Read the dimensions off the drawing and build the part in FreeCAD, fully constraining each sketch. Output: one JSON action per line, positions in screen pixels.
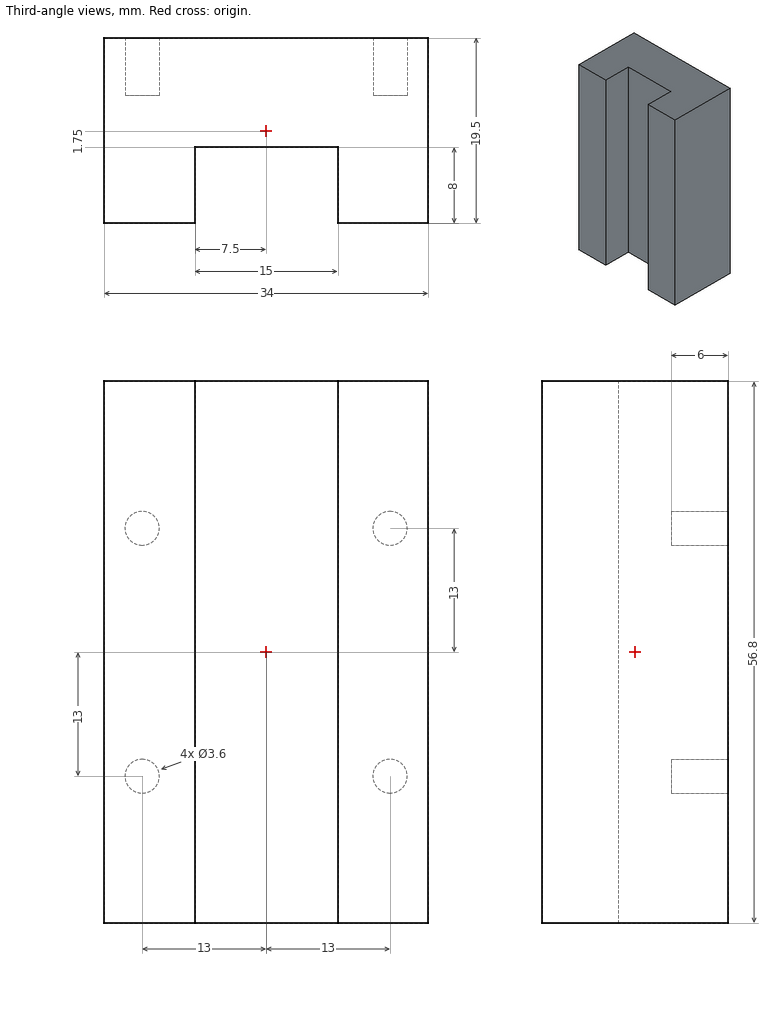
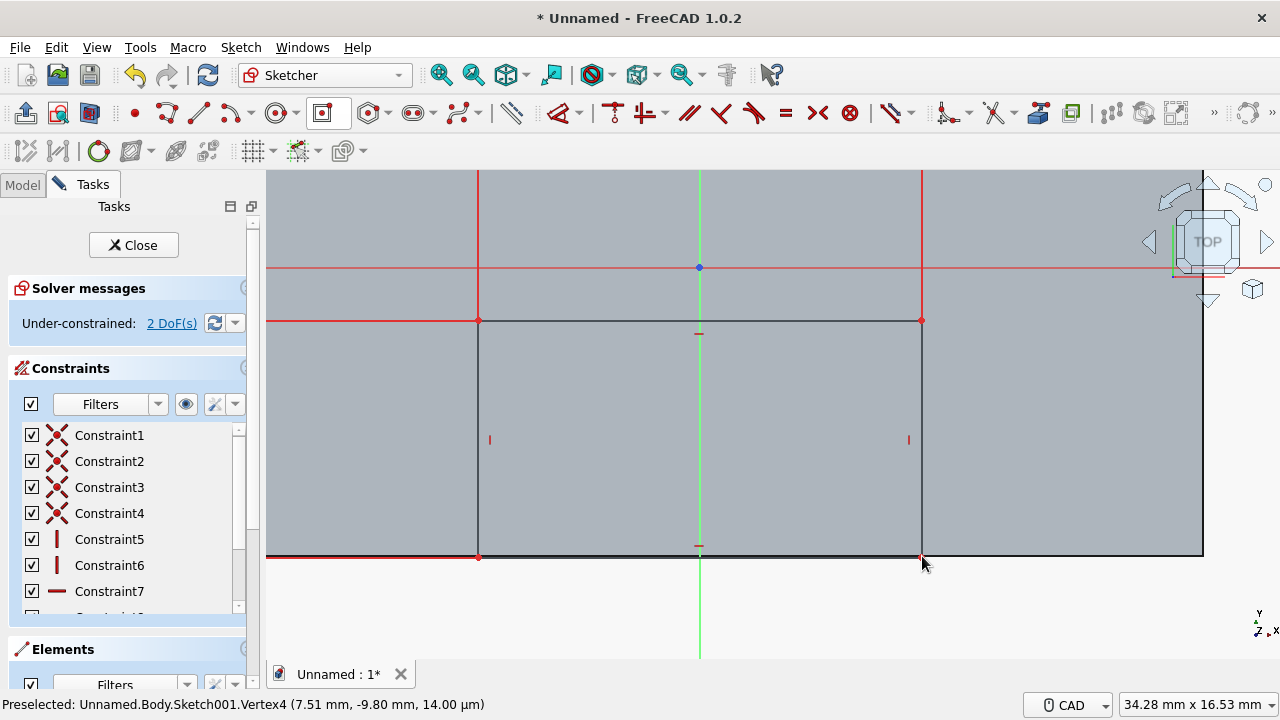
{"action": "left_click", "coordinate": [478, 321]}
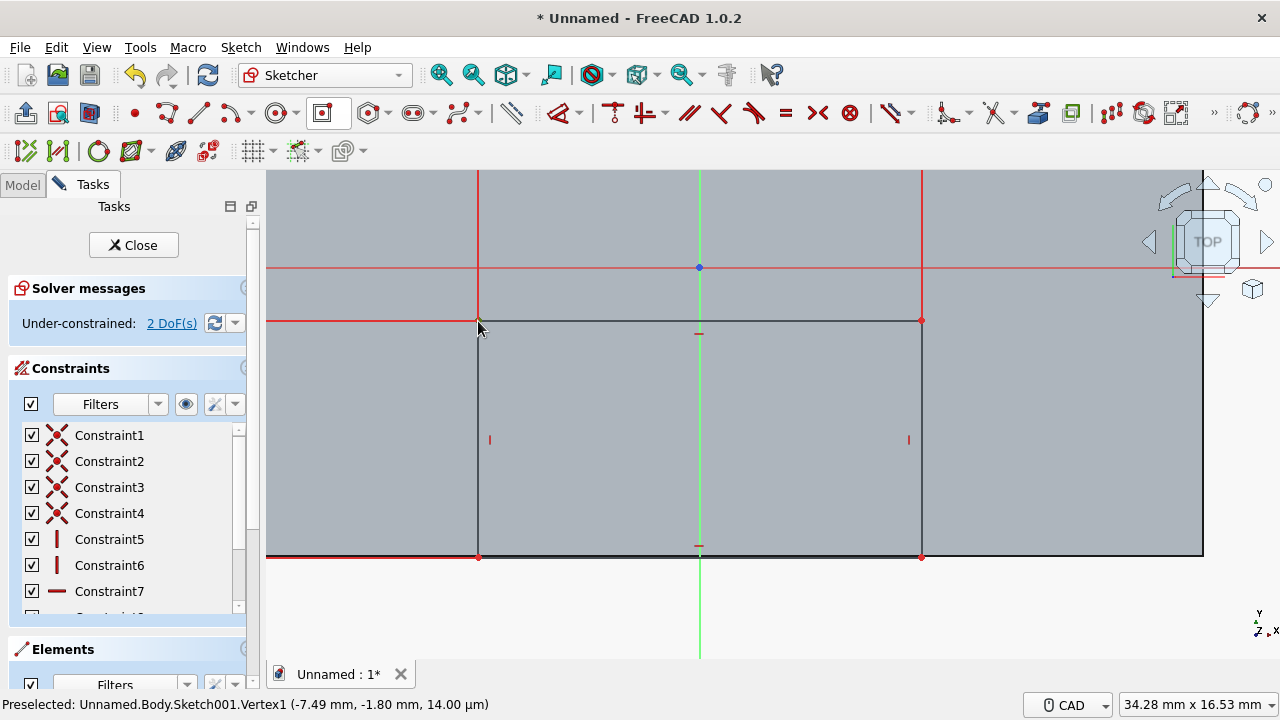
{"action": "key", "text": "l"}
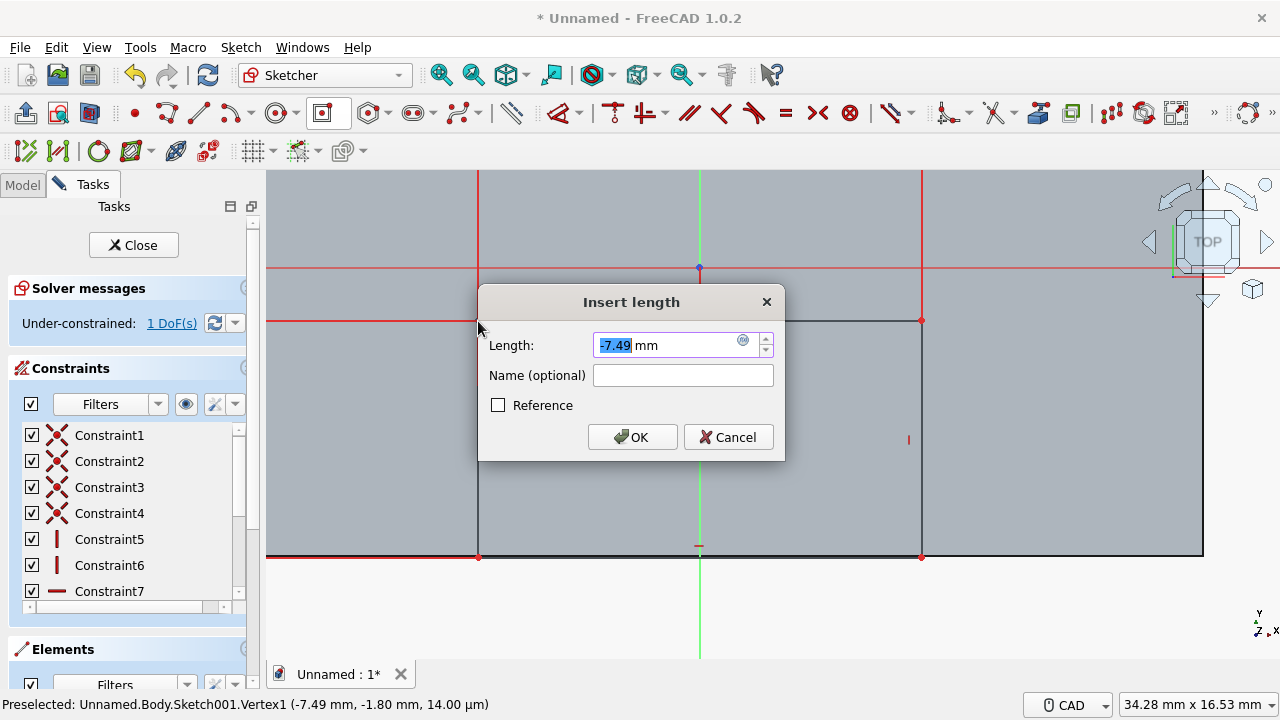
{"action": "type", "text": "-7.5"}
{"action": "key", "text": "Return"}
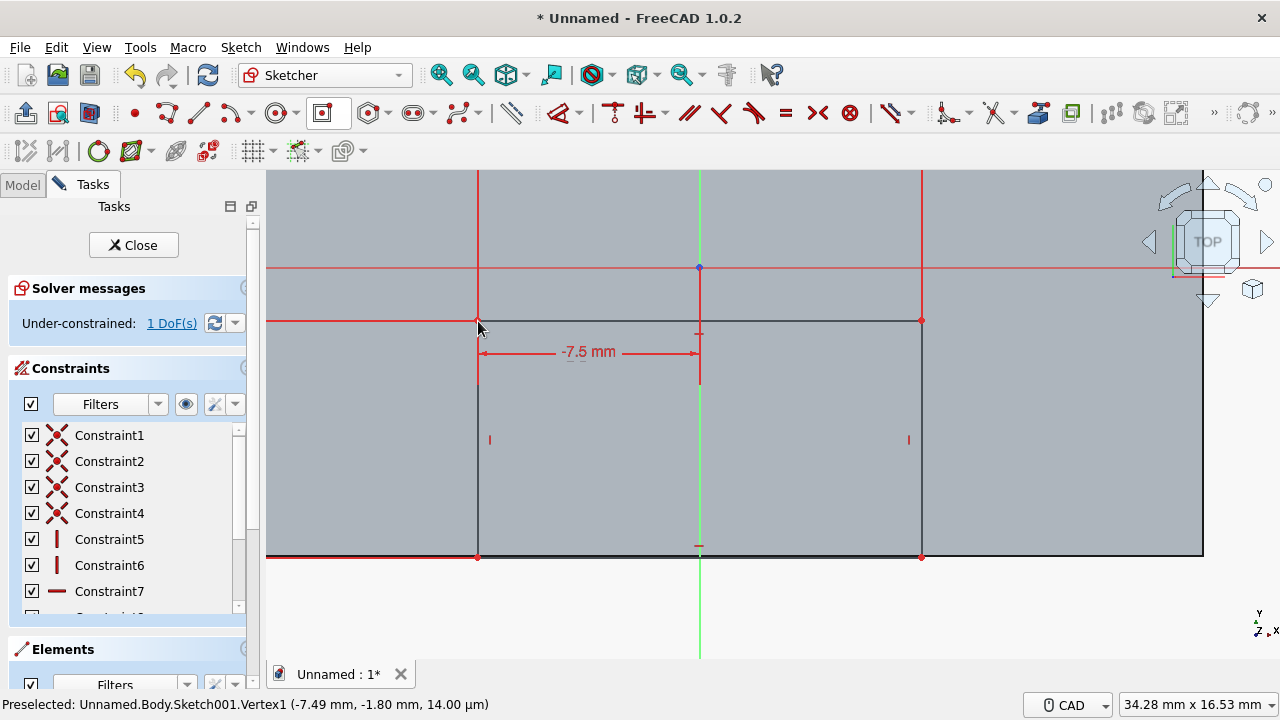
{"action": "left_click", "coordinate": [478, 321]}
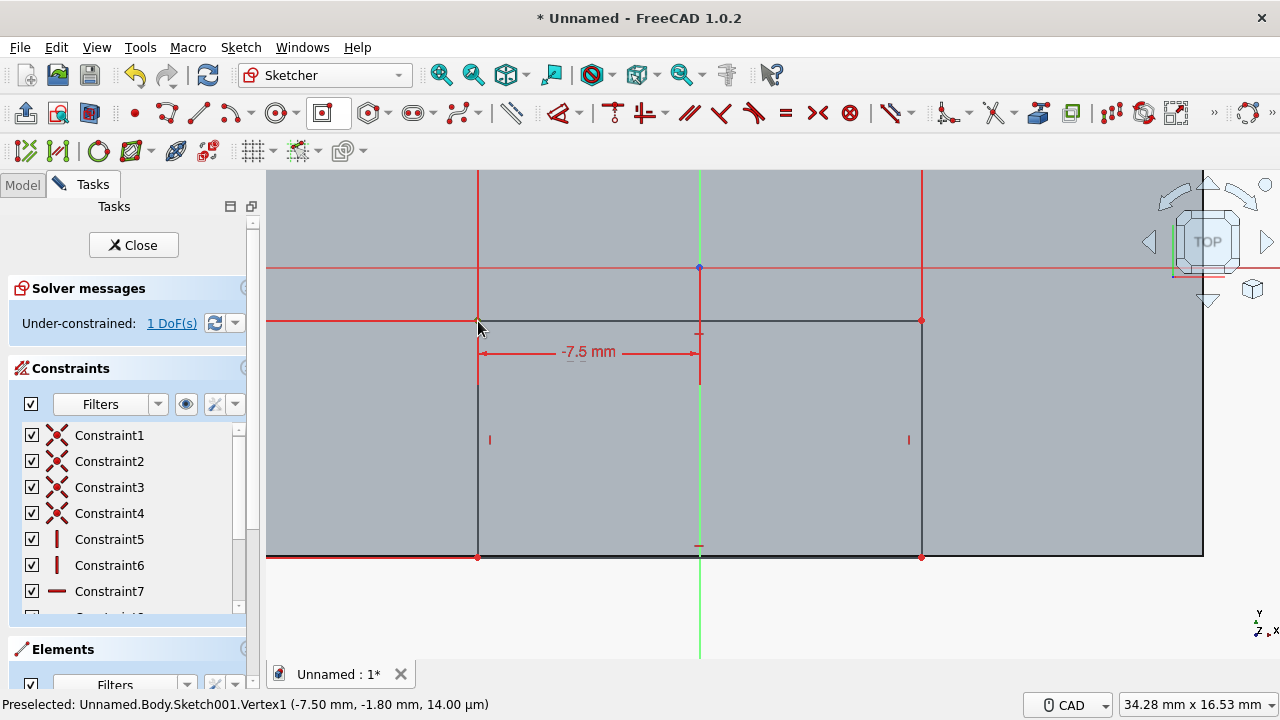
{"action": "left_click", "coordinate": [582, 114]}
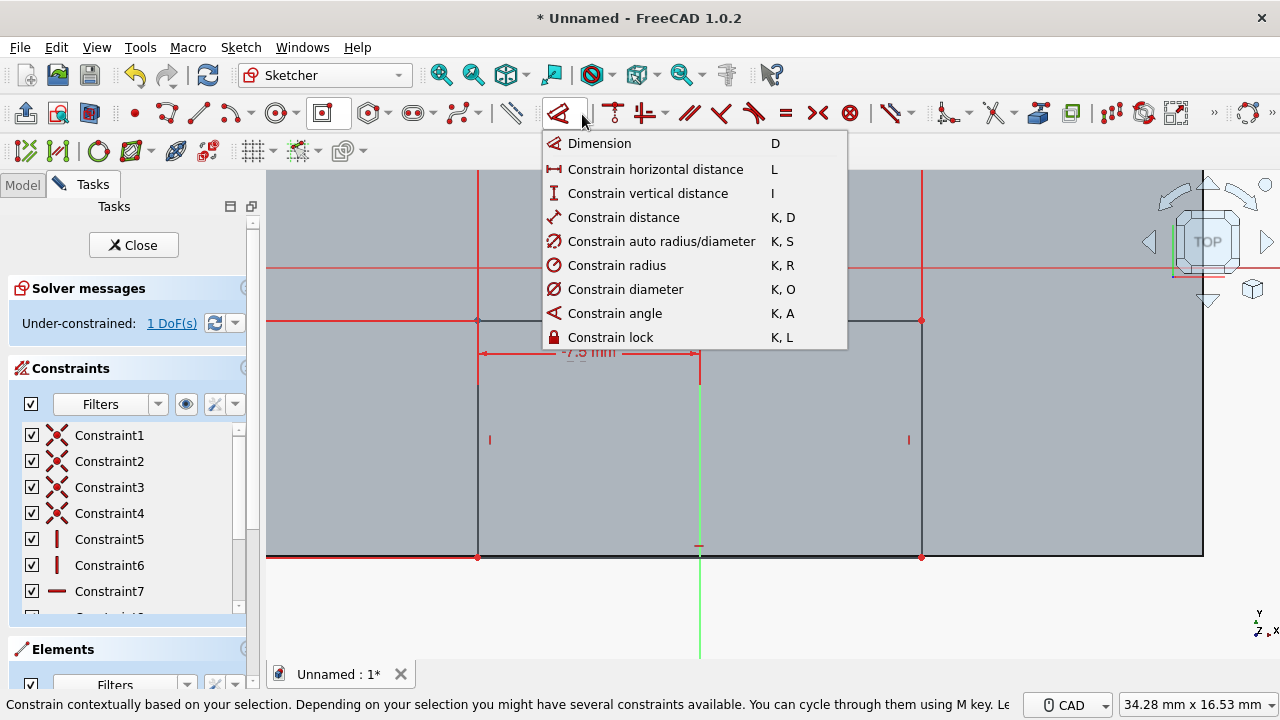
{"action": "left_click", "coordinate": [695, 193]}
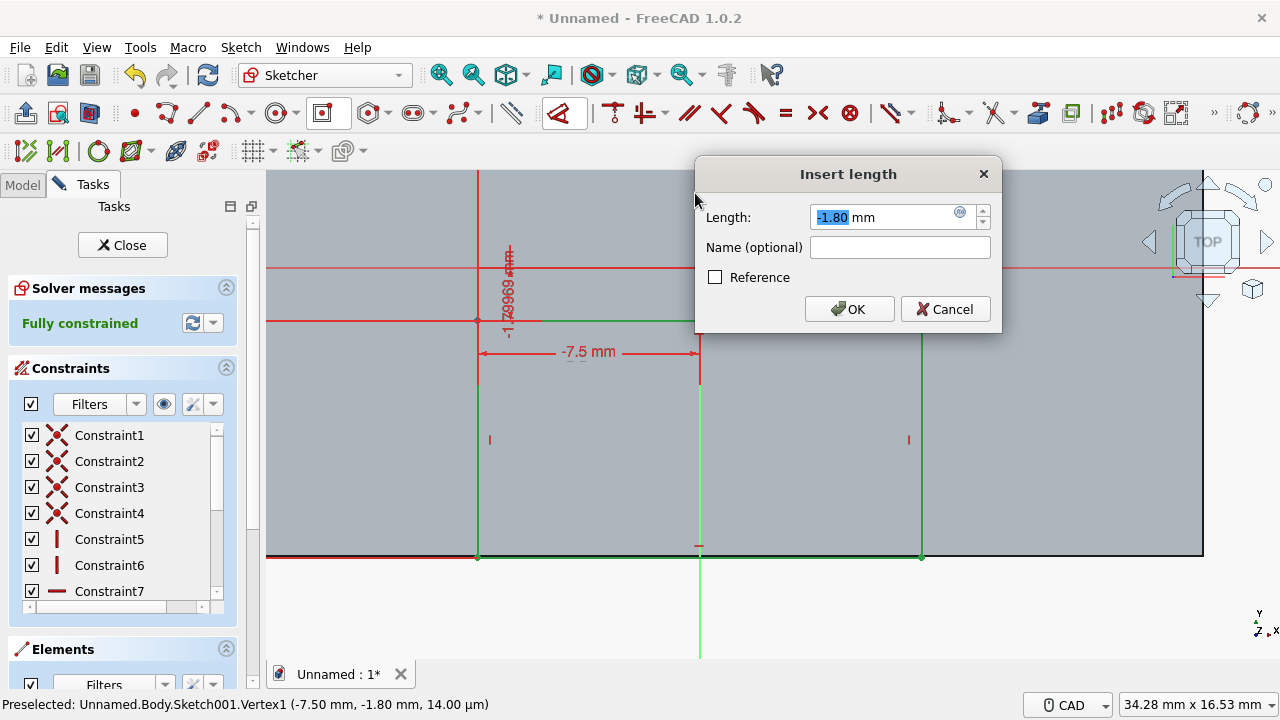
{"action": "type", "text": "-1.75"}
{"action": "key", "text": "Return"}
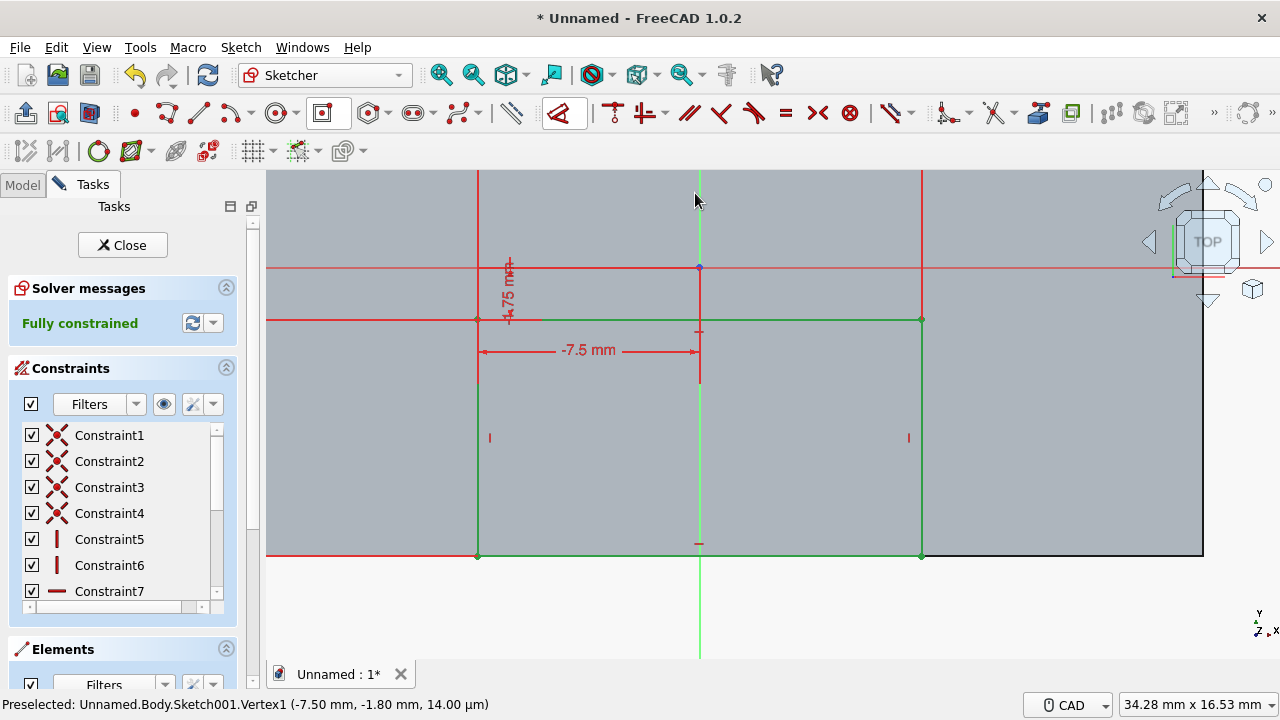
{"action": "left_click", "coordinate": [123, 245]}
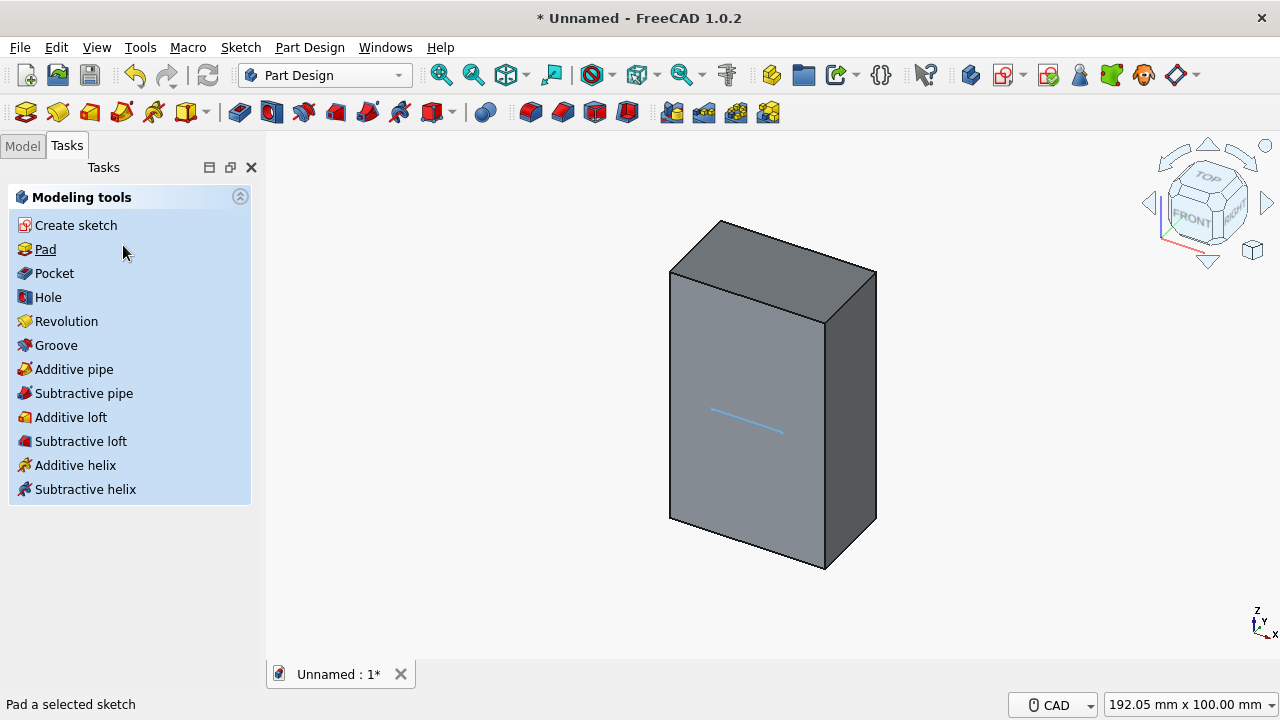
{"action": "left_click", "coordinate": [240, 112]}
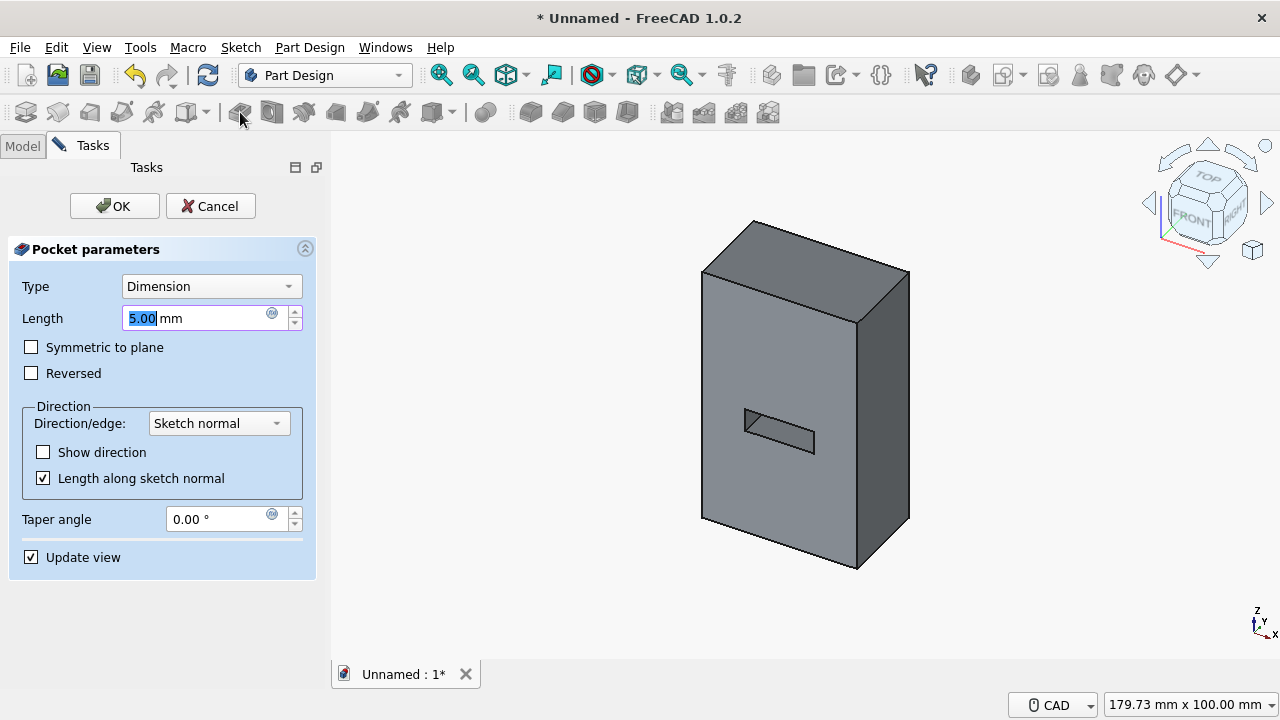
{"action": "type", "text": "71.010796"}
{"action": "key", "text": "Tab"}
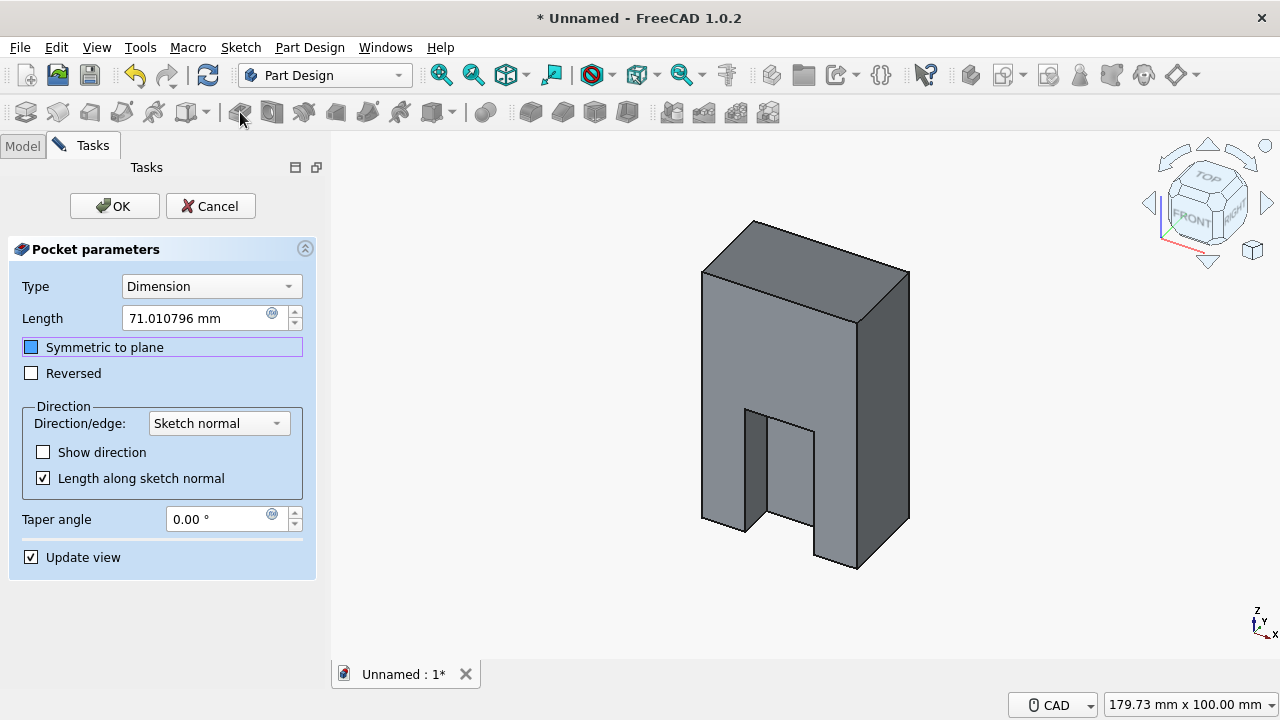
{"action": "left_click", "coordinate": [30, 347]}